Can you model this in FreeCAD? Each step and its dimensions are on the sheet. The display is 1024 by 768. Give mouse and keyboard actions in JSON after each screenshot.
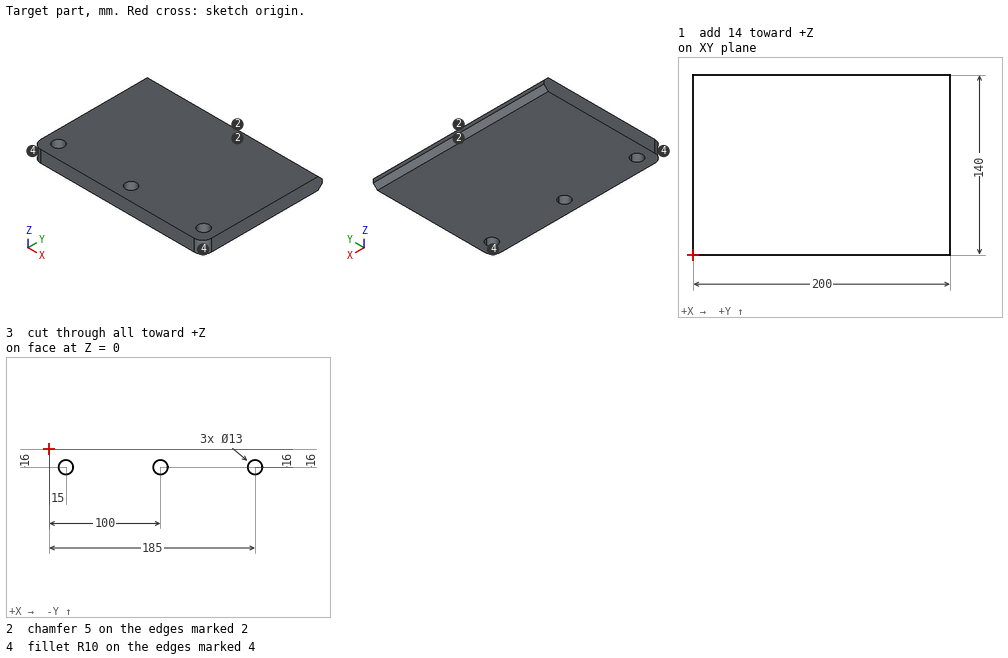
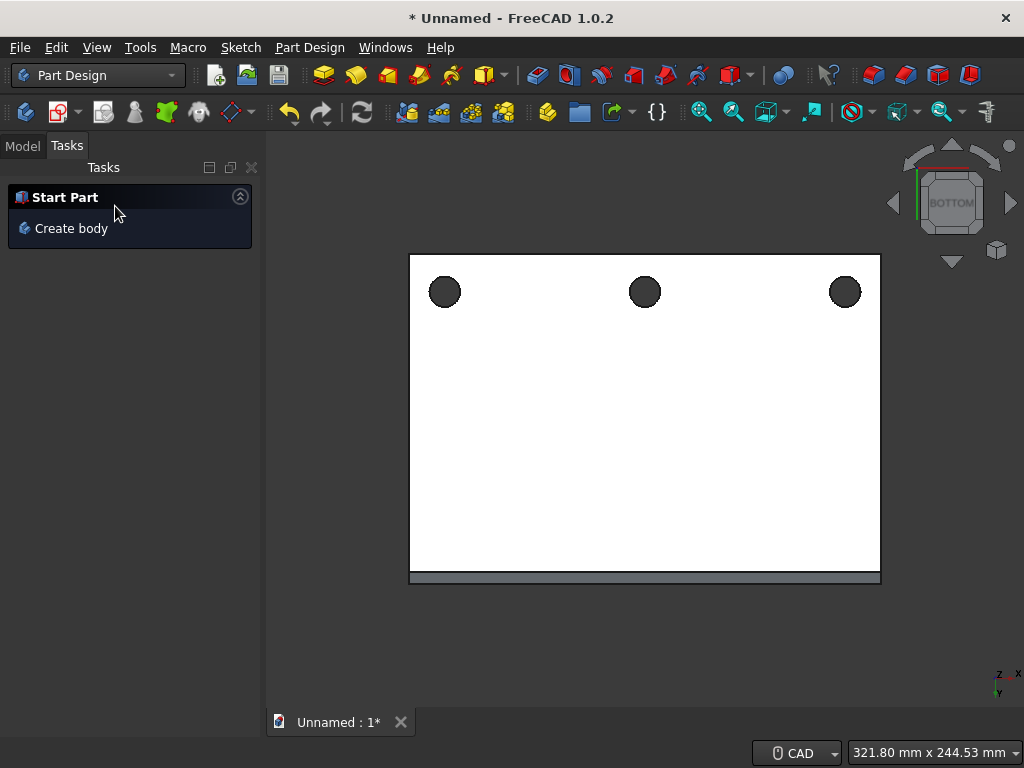
{"action": "key", "text": "0"}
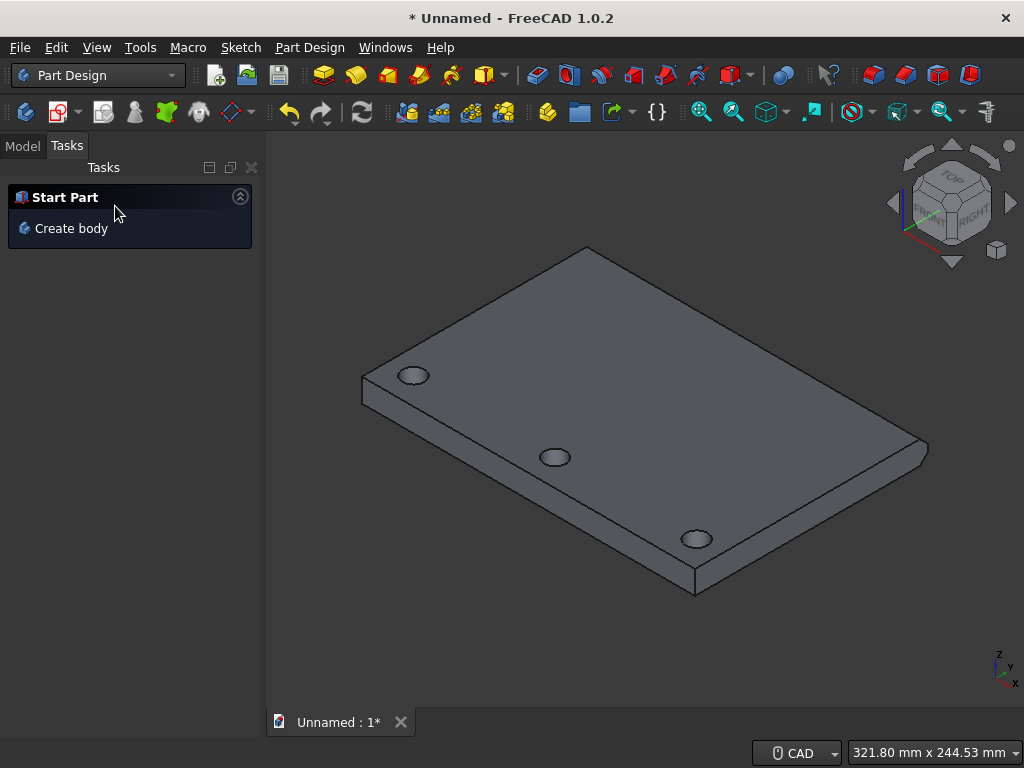
{"action": "left_click", "coordinate": [695, 581]}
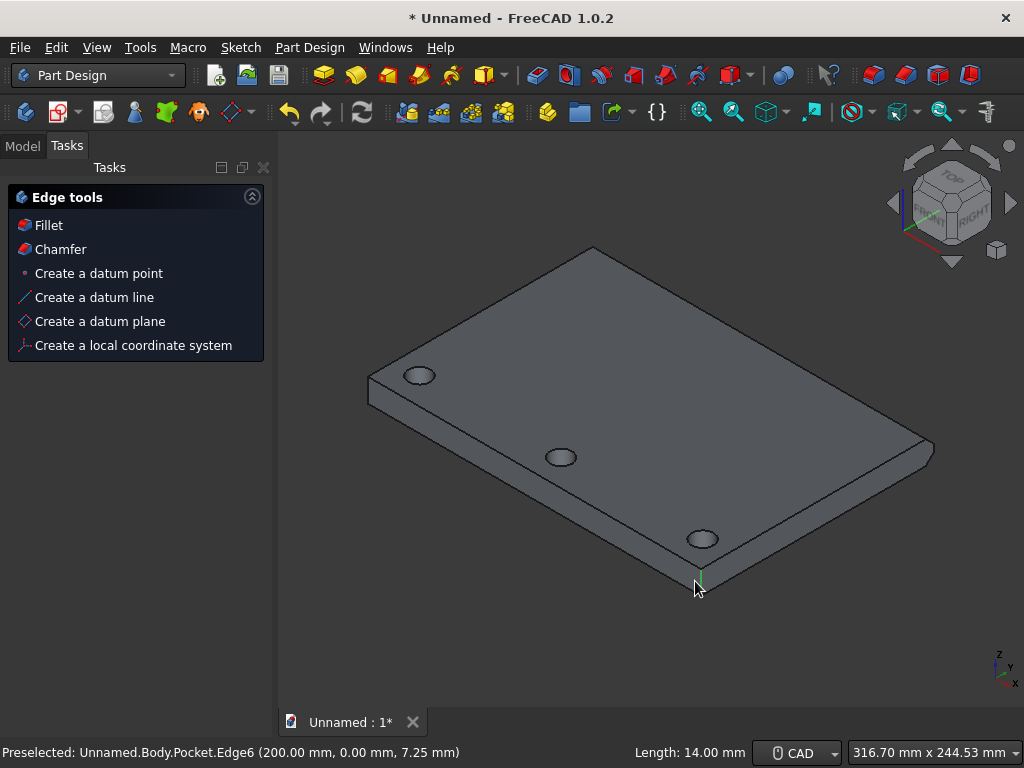
{"action": "key", "text": "2"}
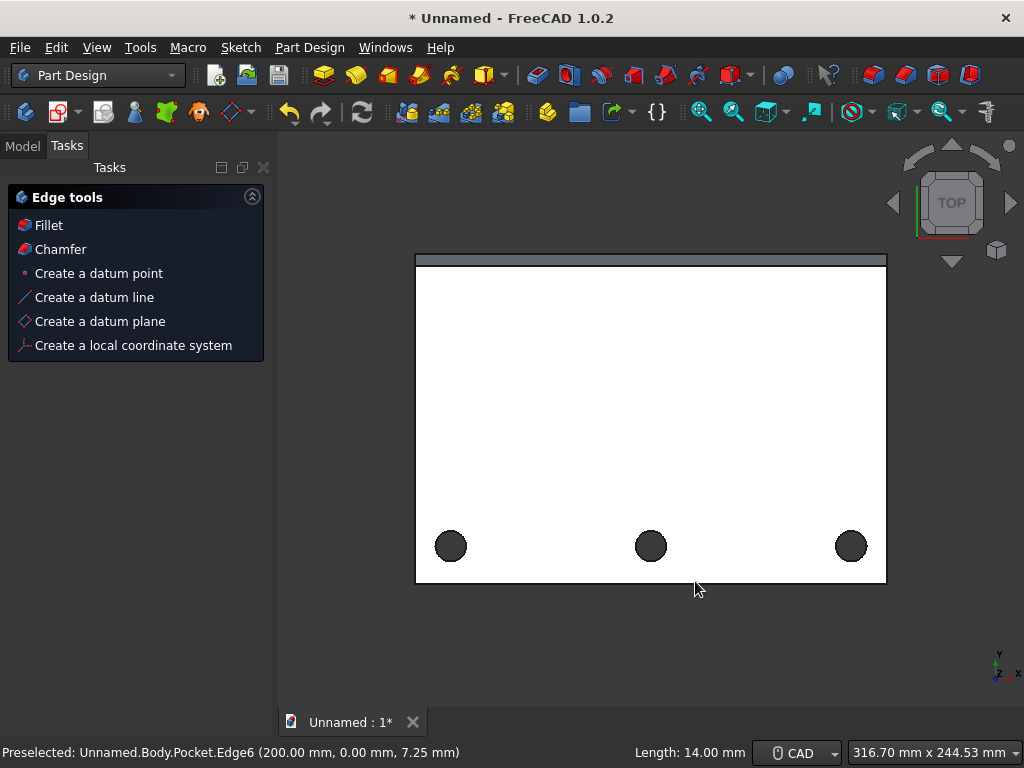
{"action": "key", "text": "1"}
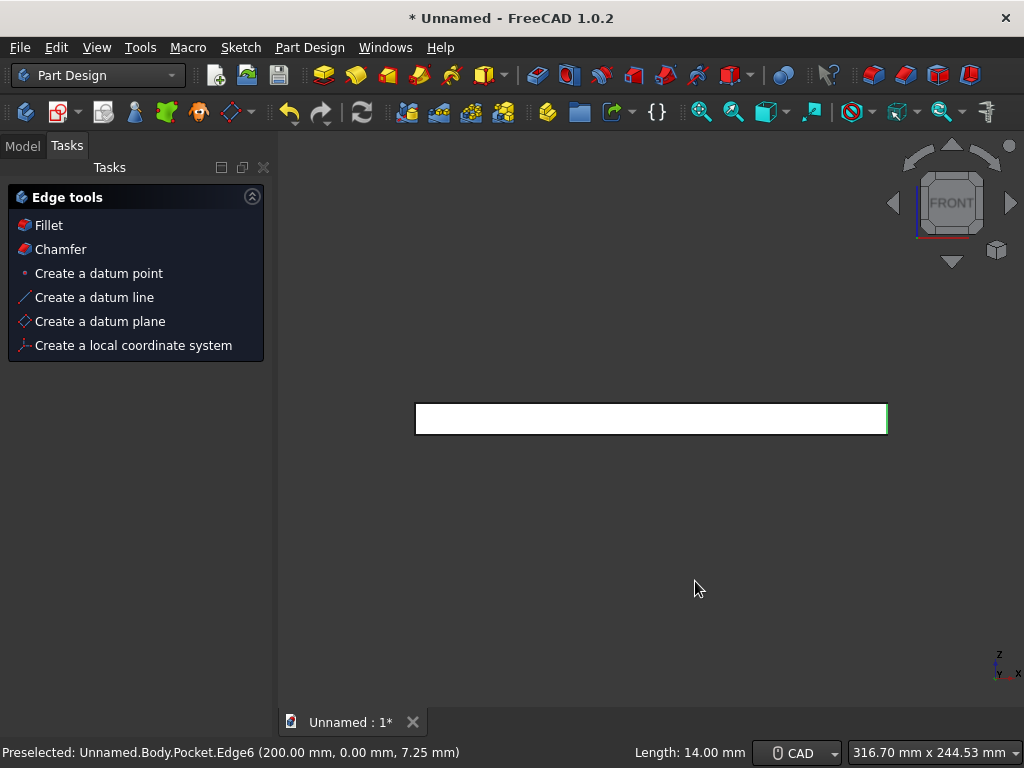
{"action": "left_click", "coordinate": [415, 418], "text": "ctrl"}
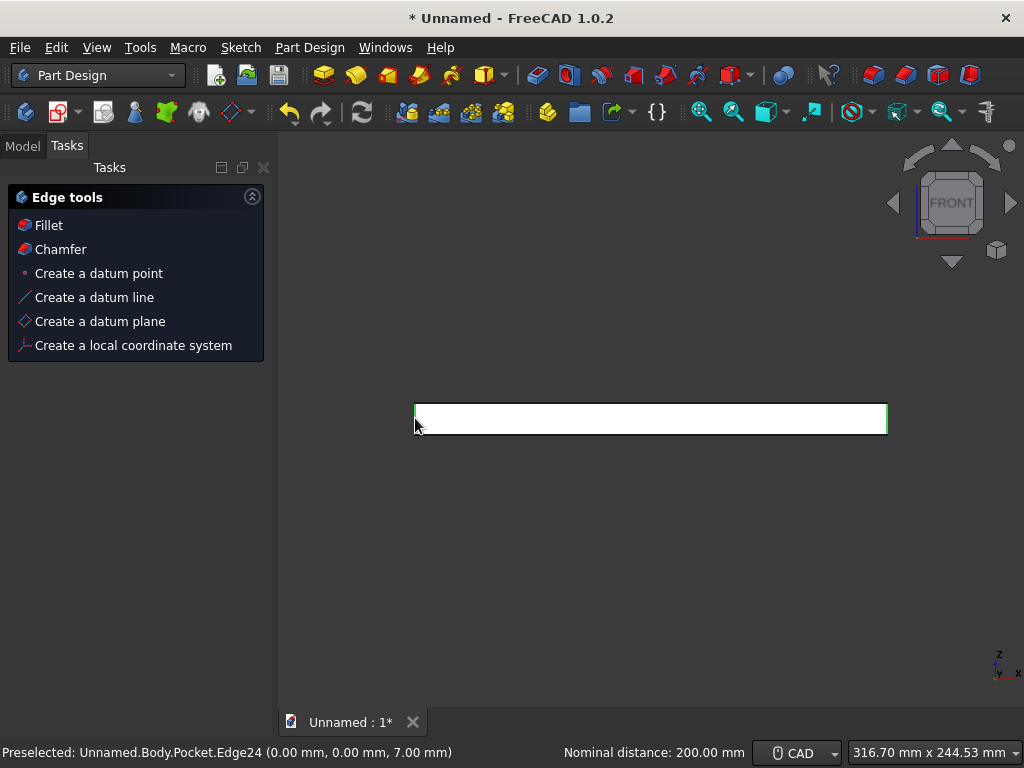
{"action": "left_click", "coordinate": [874, 76]}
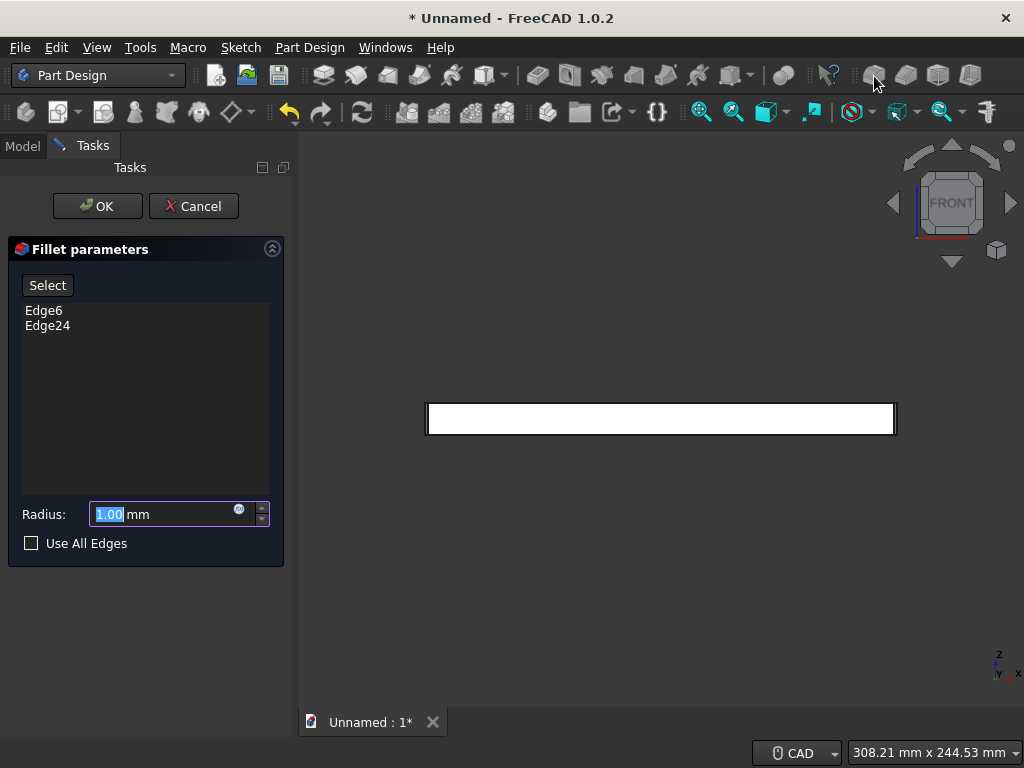
{"action": "type", "text": "10"}
{"action": "key", "text": "Tab"}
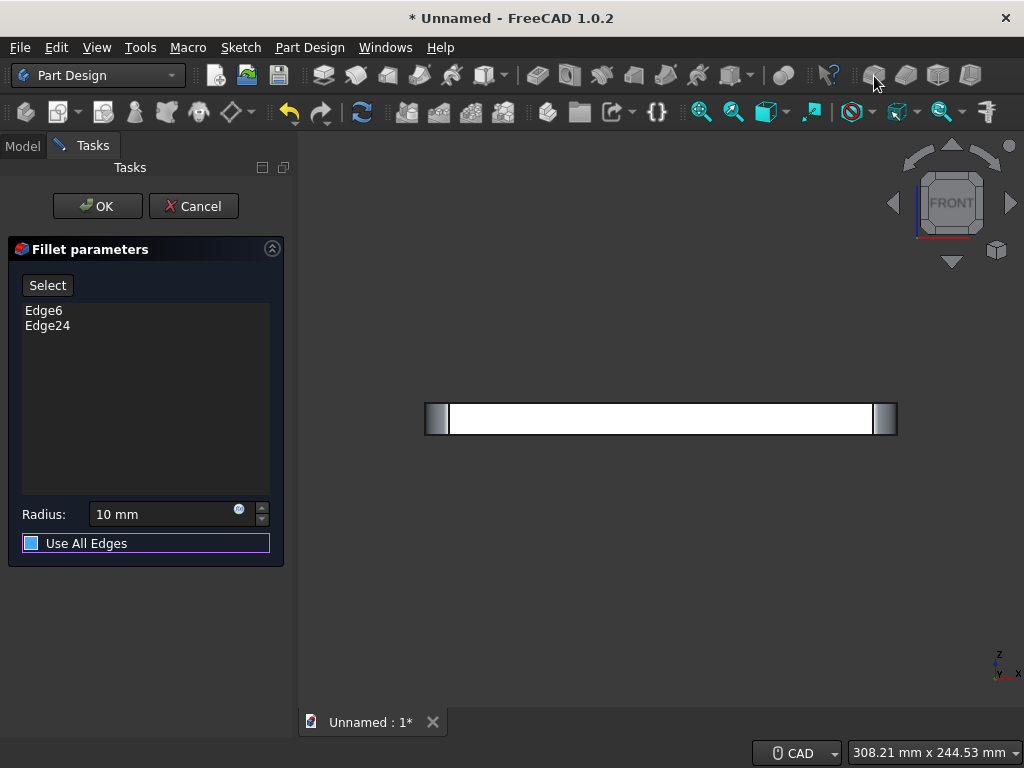
{"action": "left_click", "coordinate": [98, 206]}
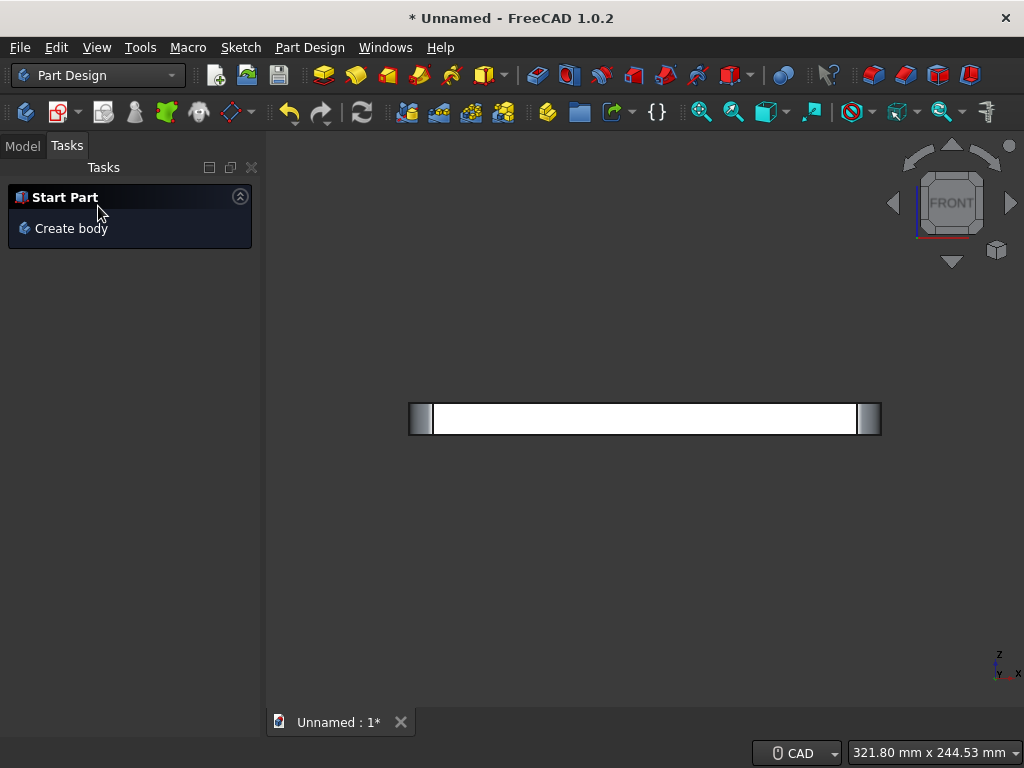
{"action": "key", "text": "0"}